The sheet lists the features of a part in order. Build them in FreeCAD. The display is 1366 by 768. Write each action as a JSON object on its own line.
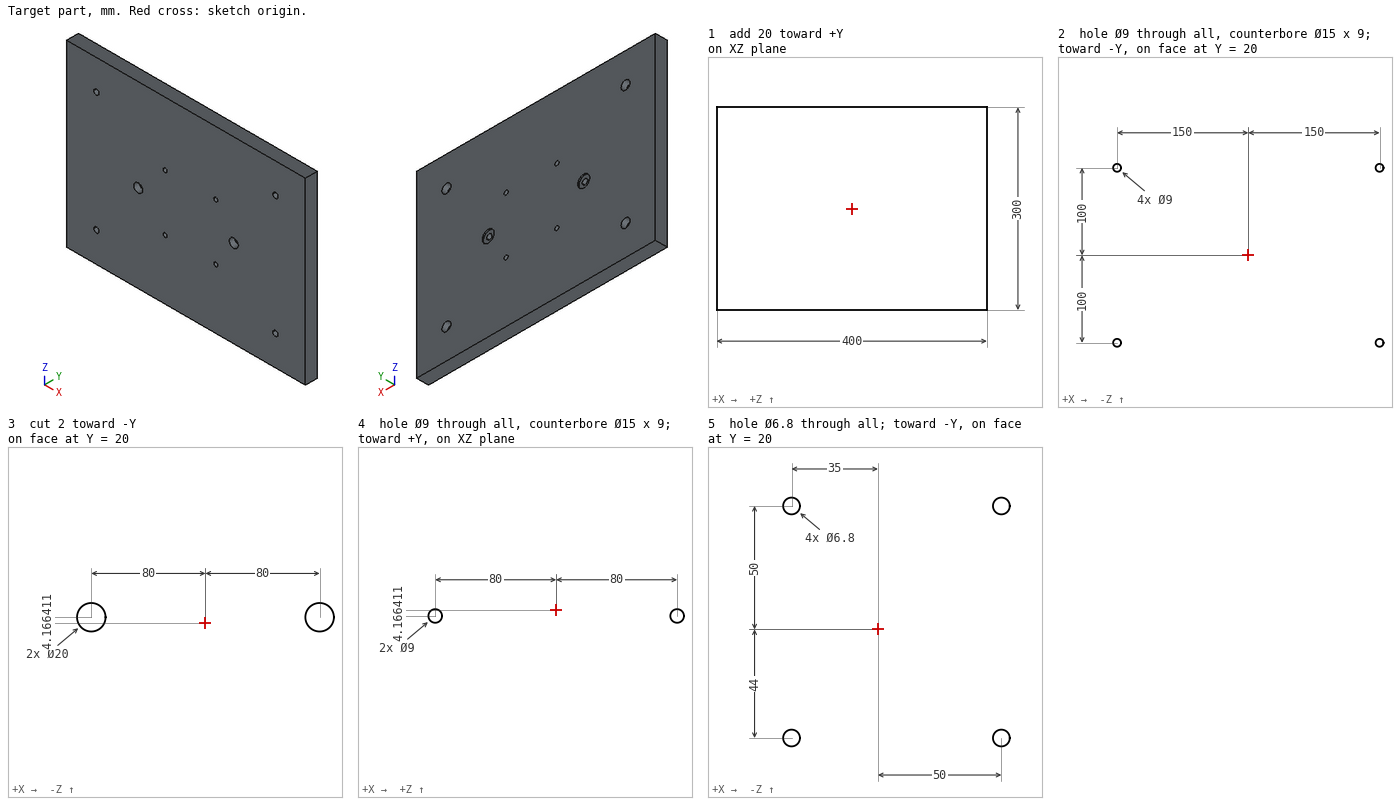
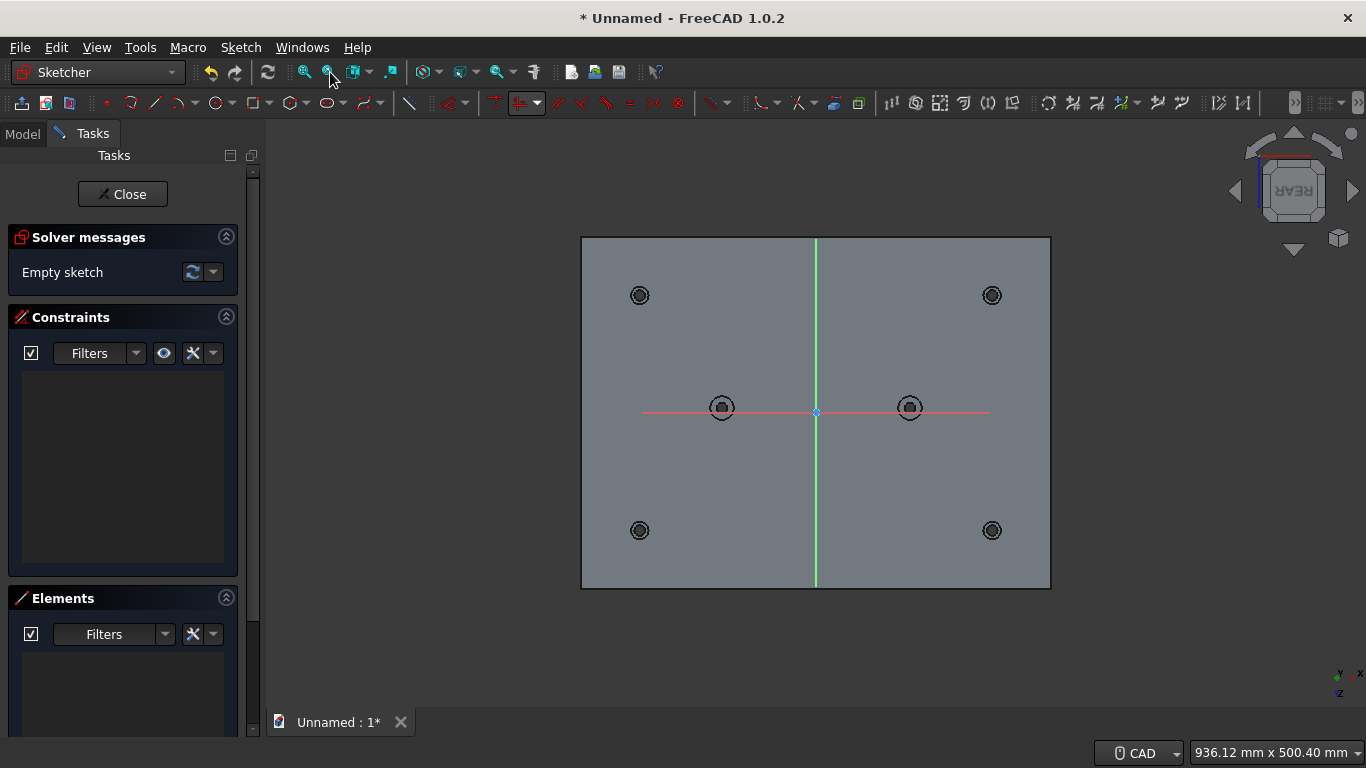
{"action": "scroll", "coordinate": [858, 408], "scroll_direction": "up", "scroll_amount": 6}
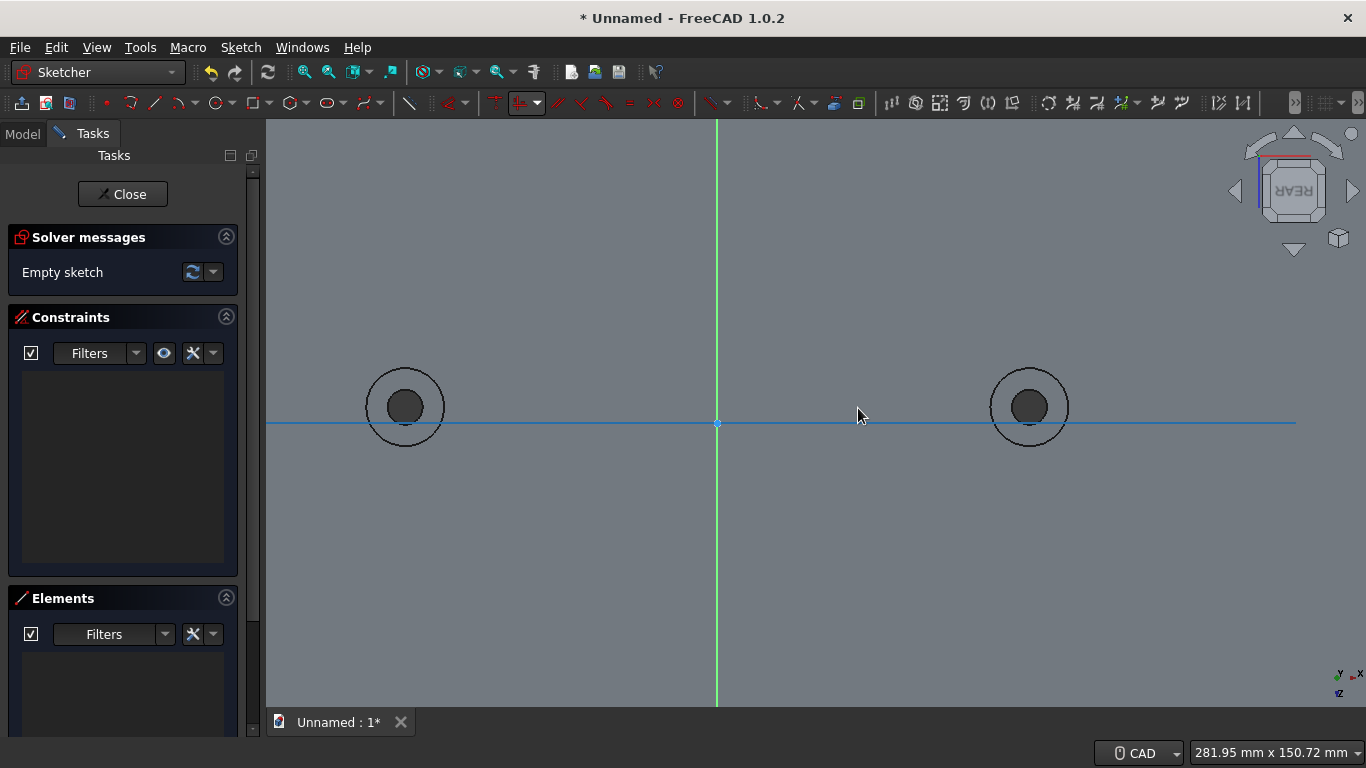
{"action": "left_click", "coordinate": [216, 104]}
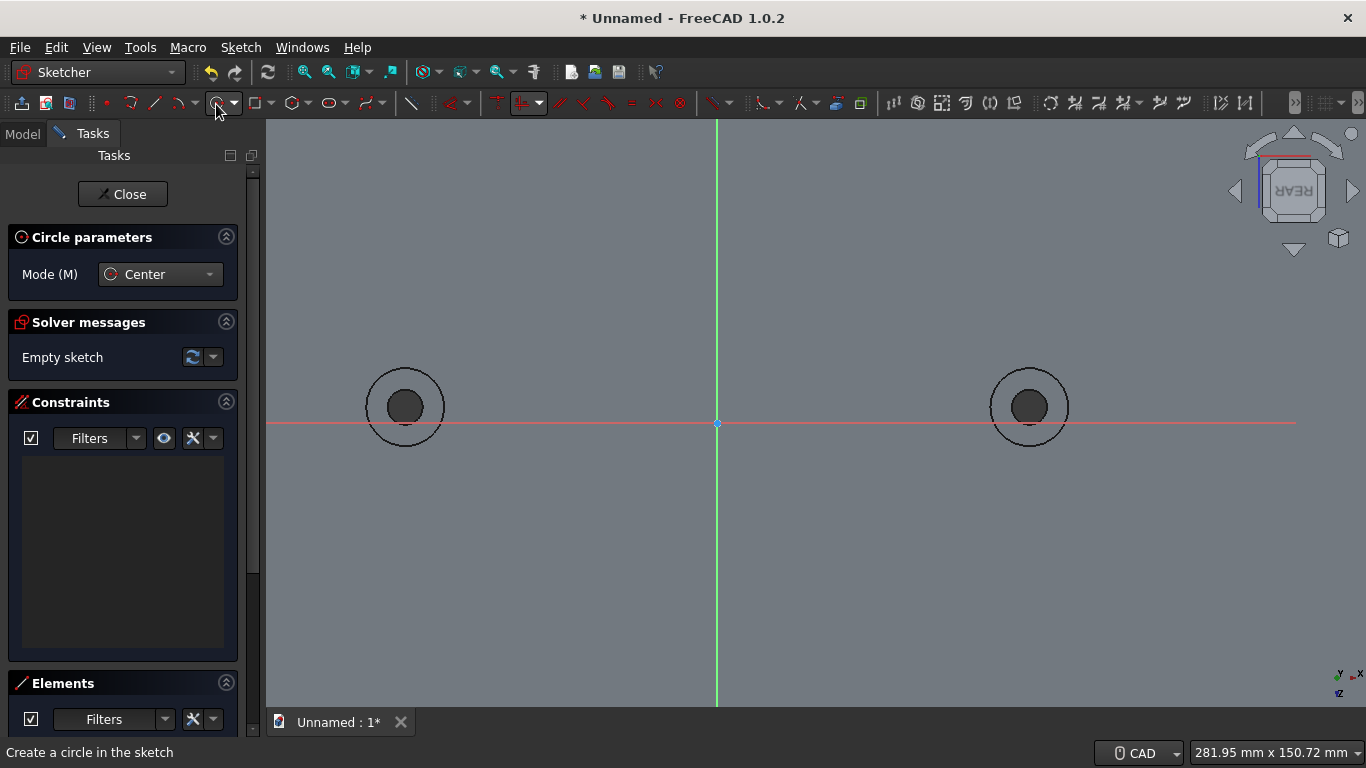
{"action": "scroll", "coordinate": [581, 228], "scroll_direction": "up", "scroll_amount": 3}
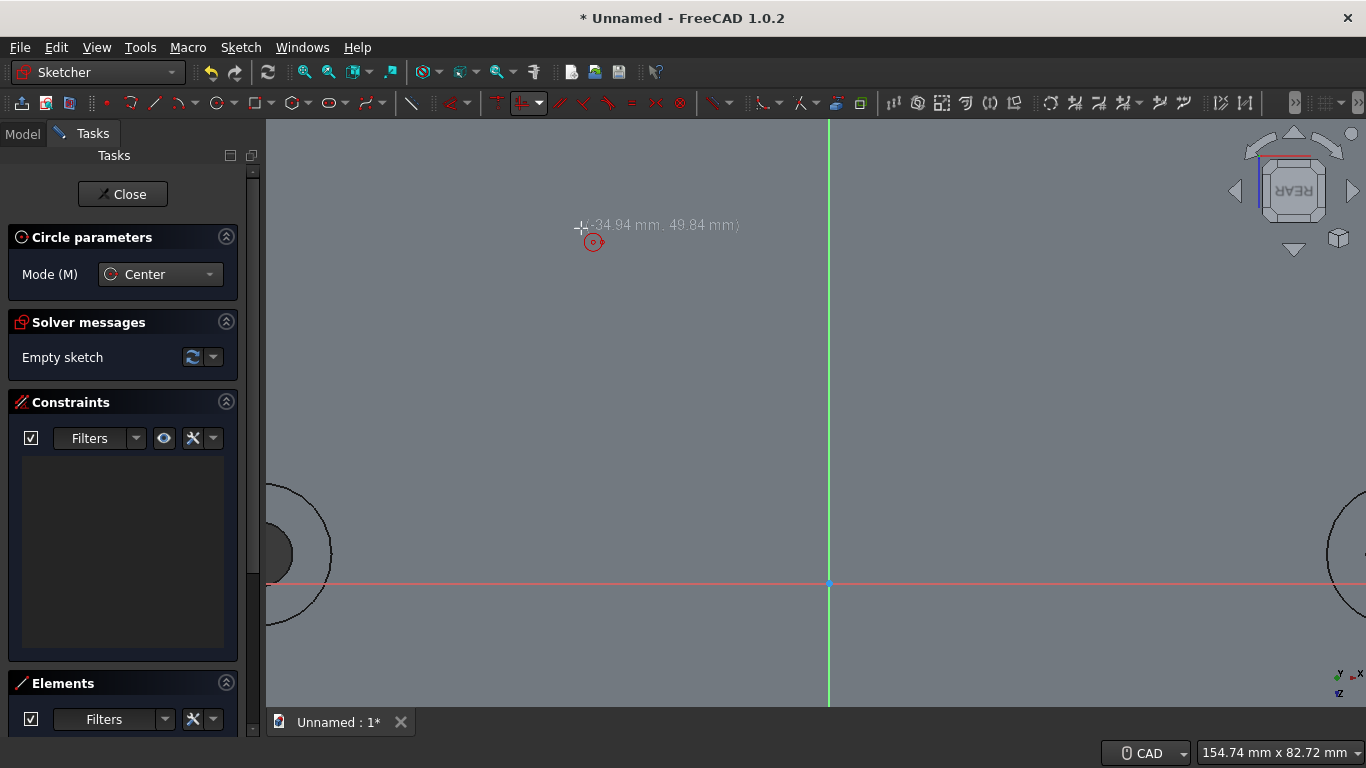
{"action": "left_click", "coordinate": [580, 229]}
{"action": "left_click", "coordinate": [597, 211]}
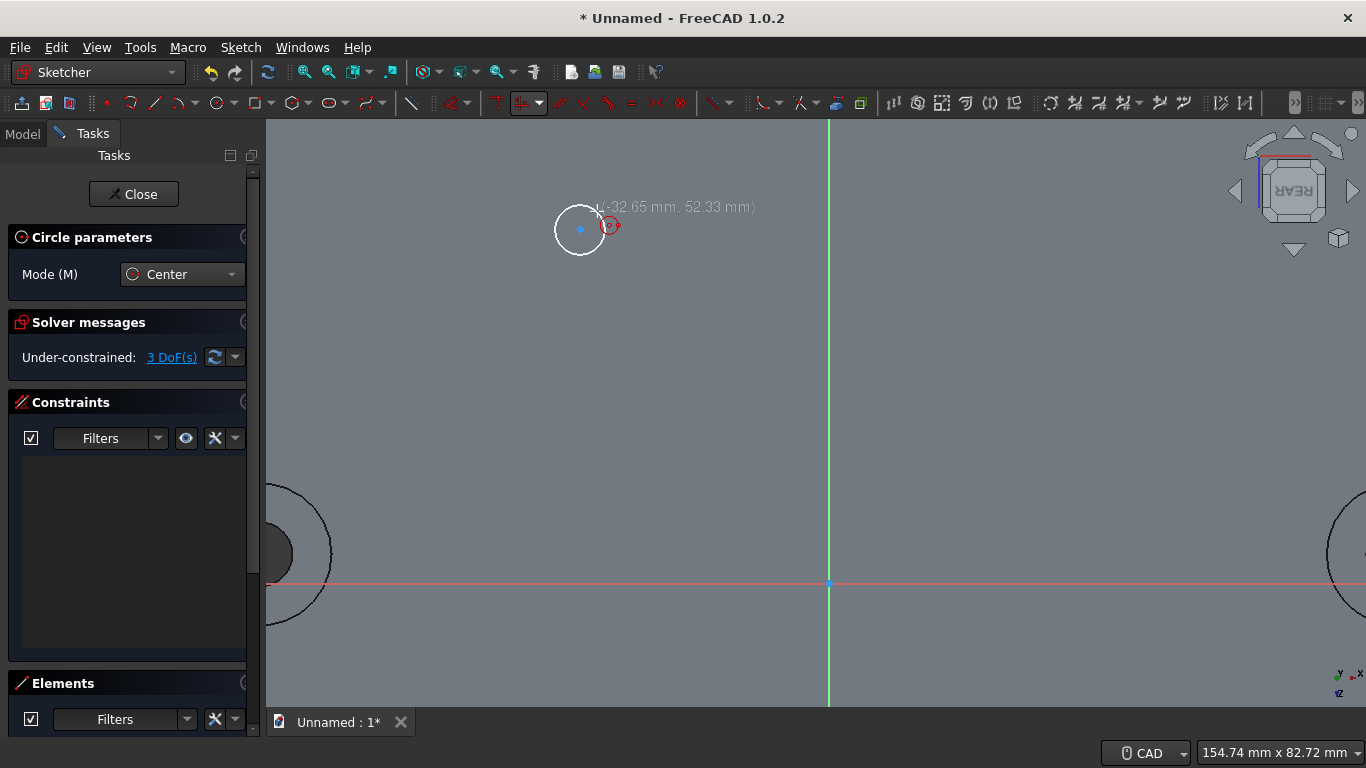
{"action": "scroll", "coordinate": [583, 231], "scroll_direction": "down", "scroll_amount": 3}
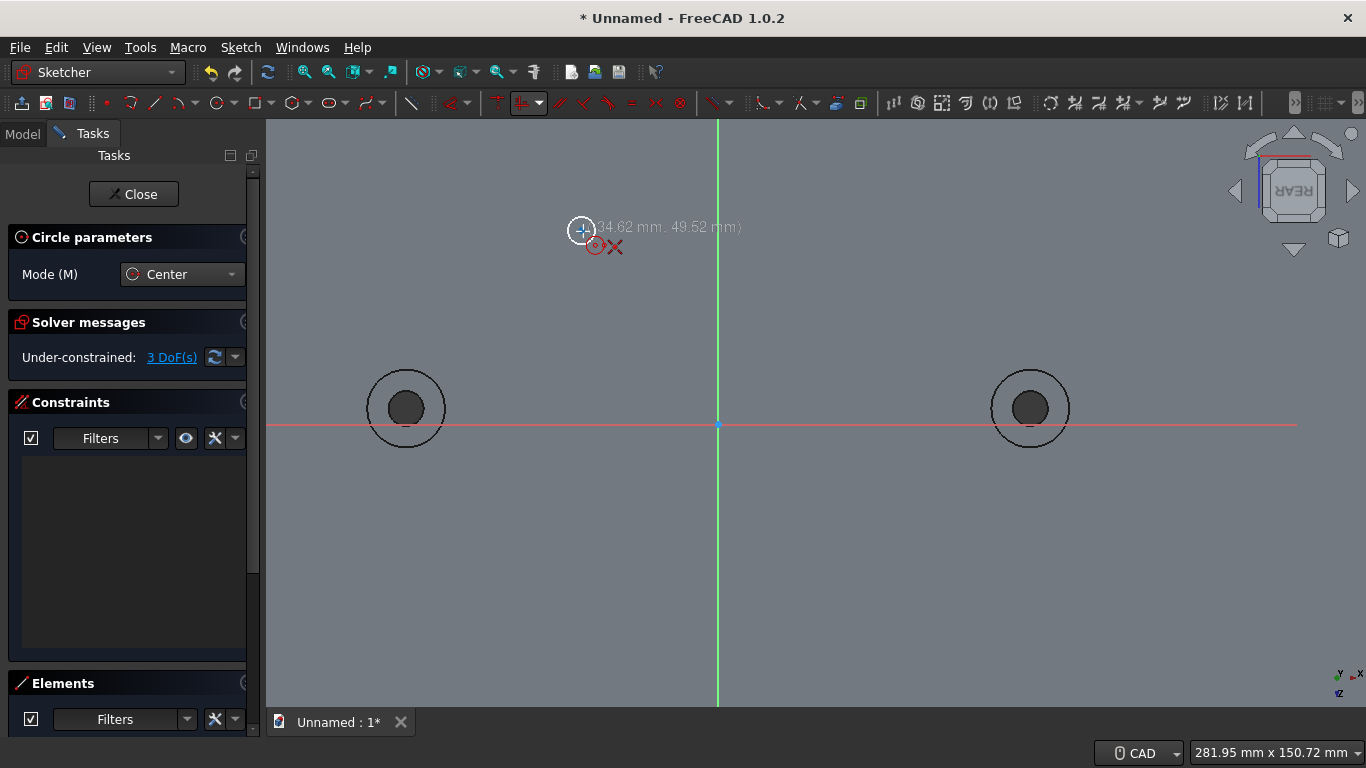
{"action": "scroll", "coordinate": [582, 596], "scroll_direction": "up", "scroll_amount": 3}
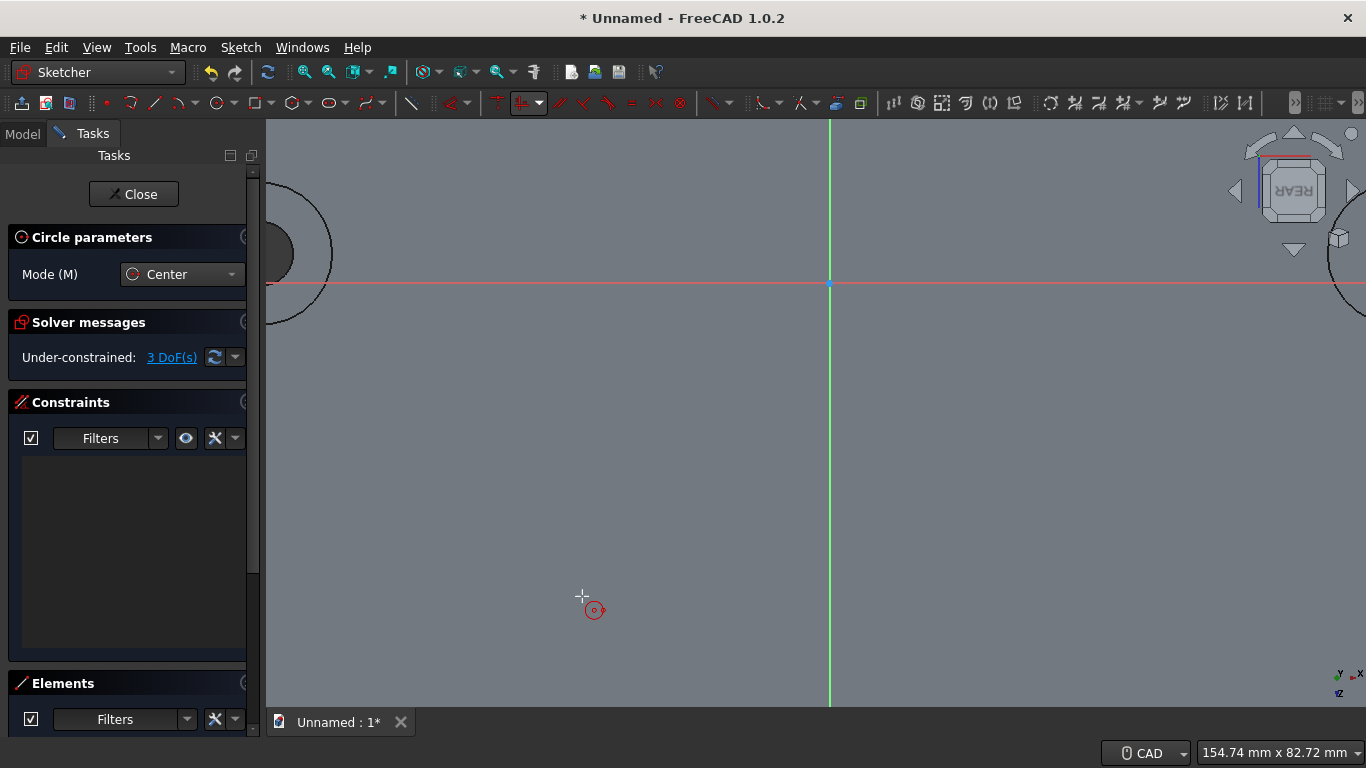
{"action": "left_click", "coordinate": [581, 596]}
{"action": "left_click", "coordinate": [598, 579]}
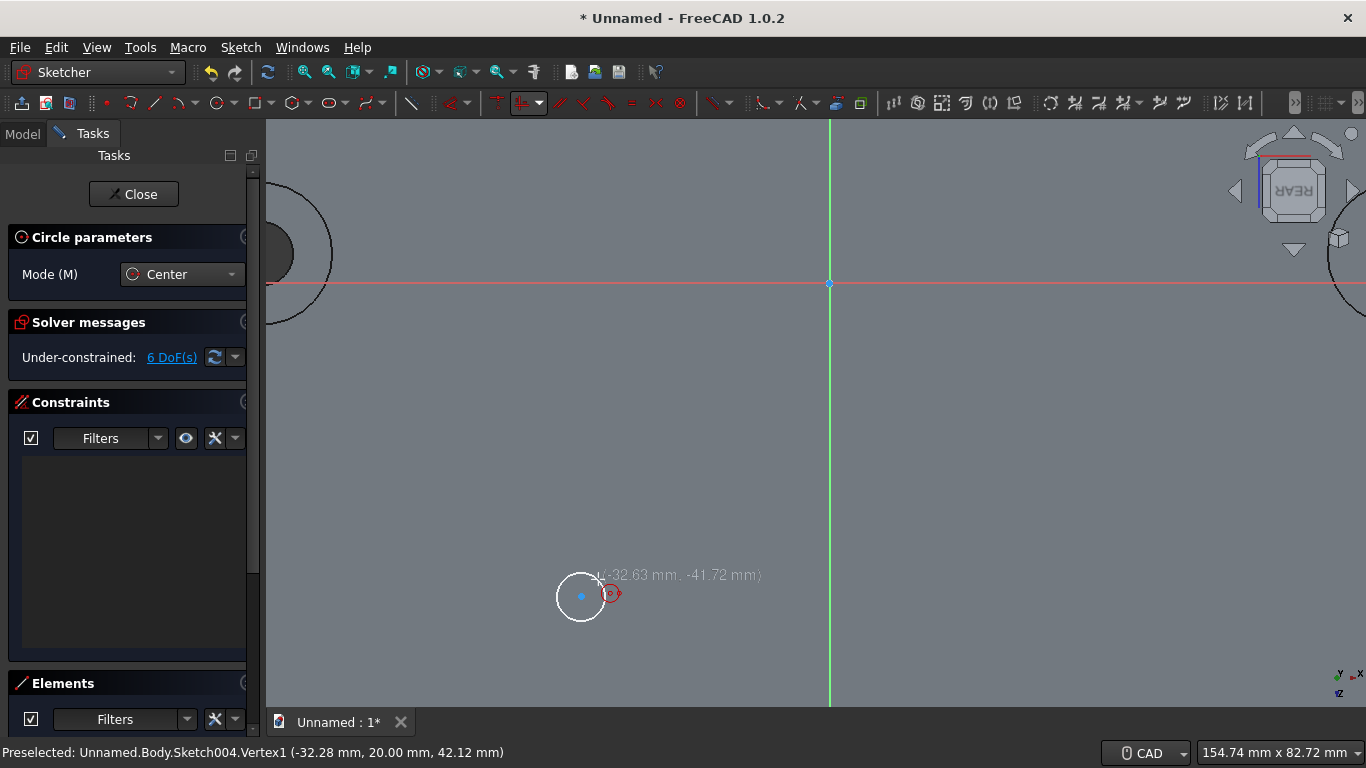
{"action": "left_click", "coordinate": [1185, 596]}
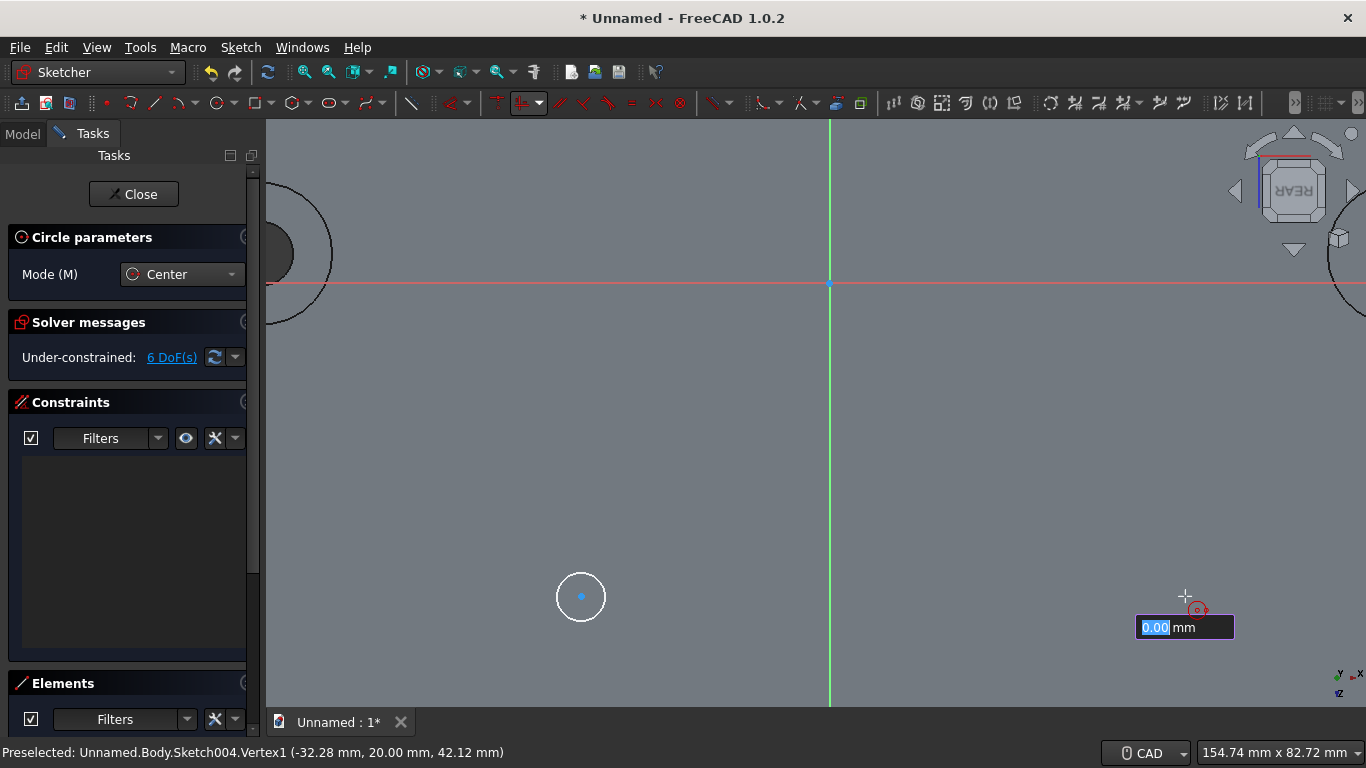
{"action": "scroll", "coordinate": [582, 597], "scroll_direction": "down", "scroll_amount": 3}